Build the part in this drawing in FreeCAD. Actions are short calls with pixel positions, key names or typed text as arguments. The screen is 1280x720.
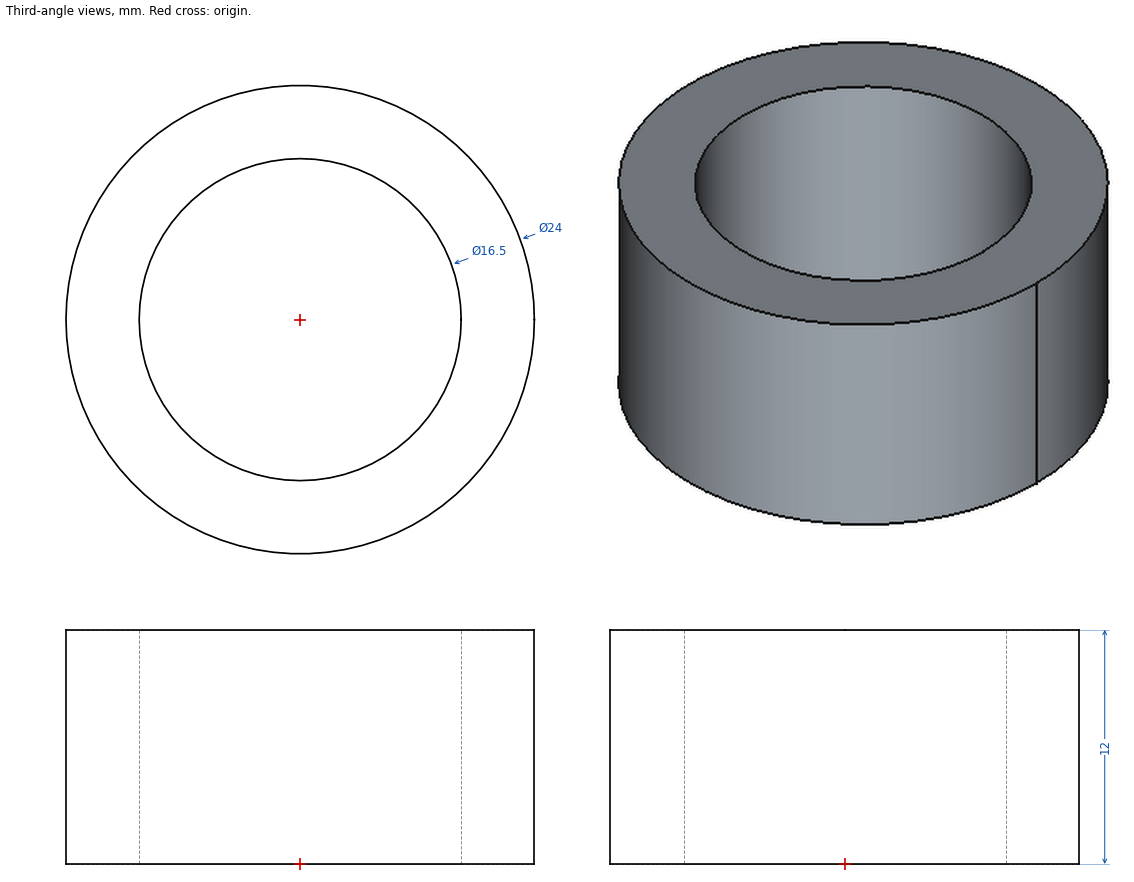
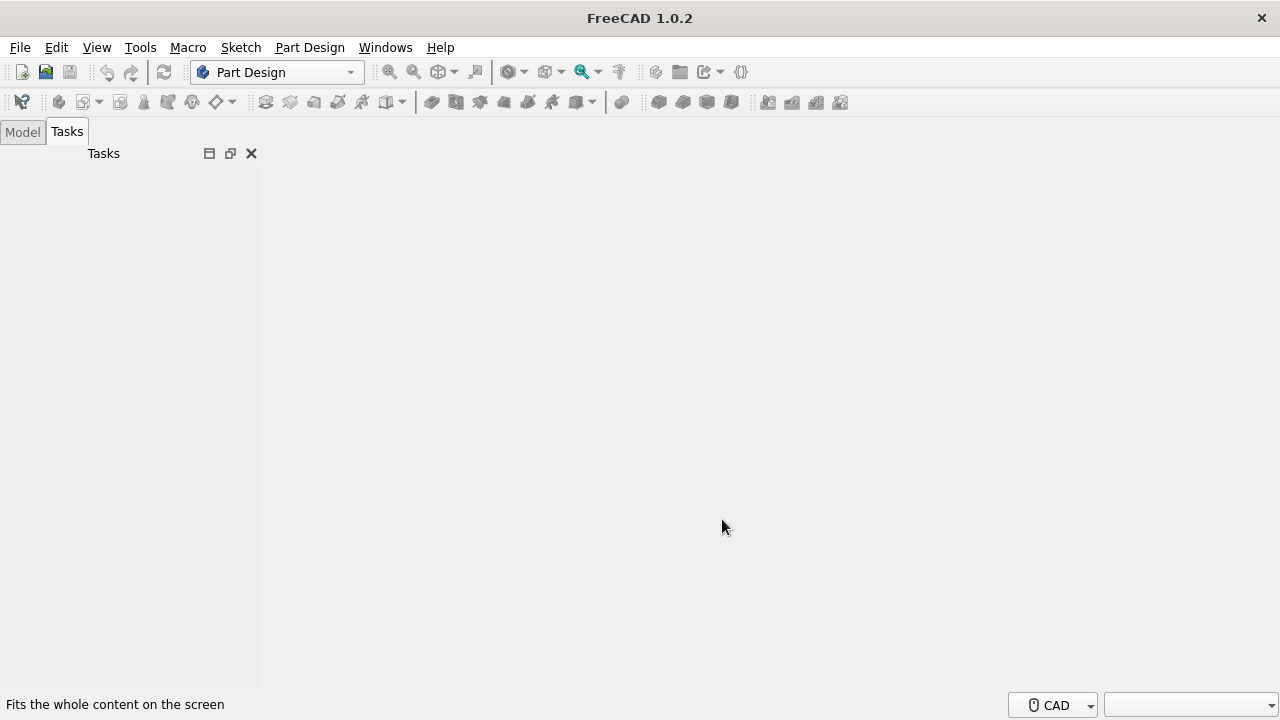
click(22, 72)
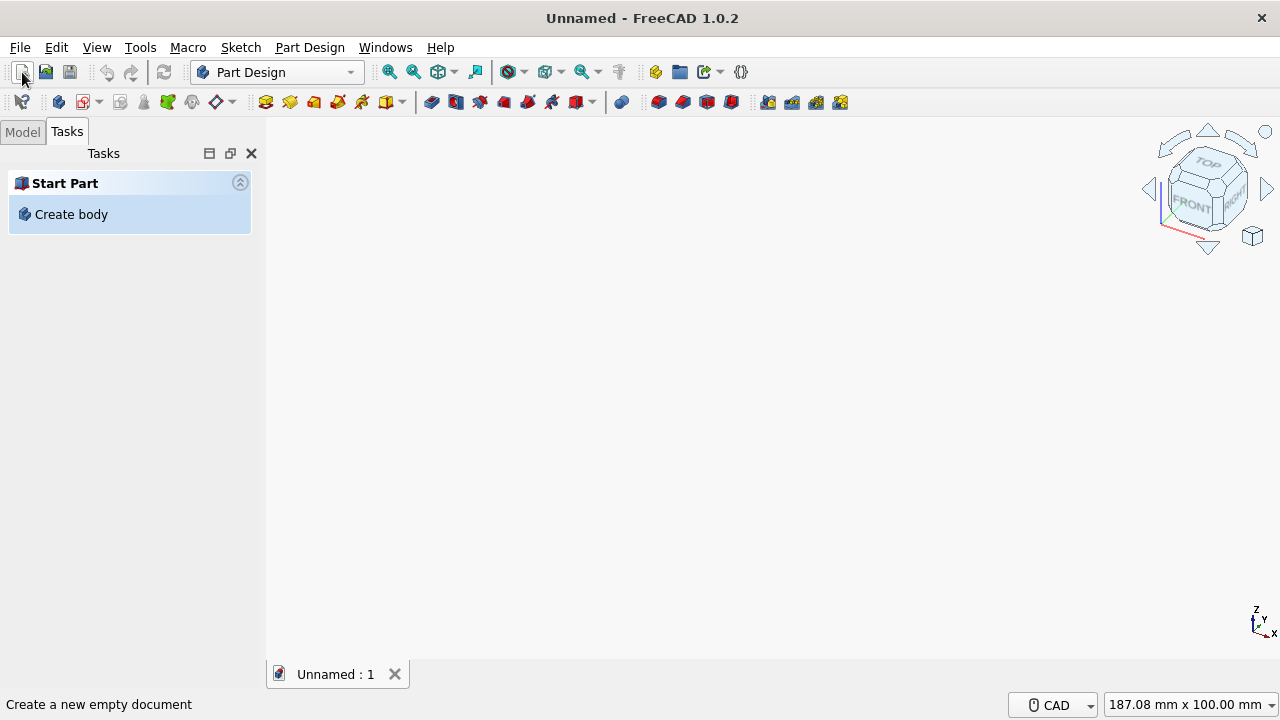
click(84, 102)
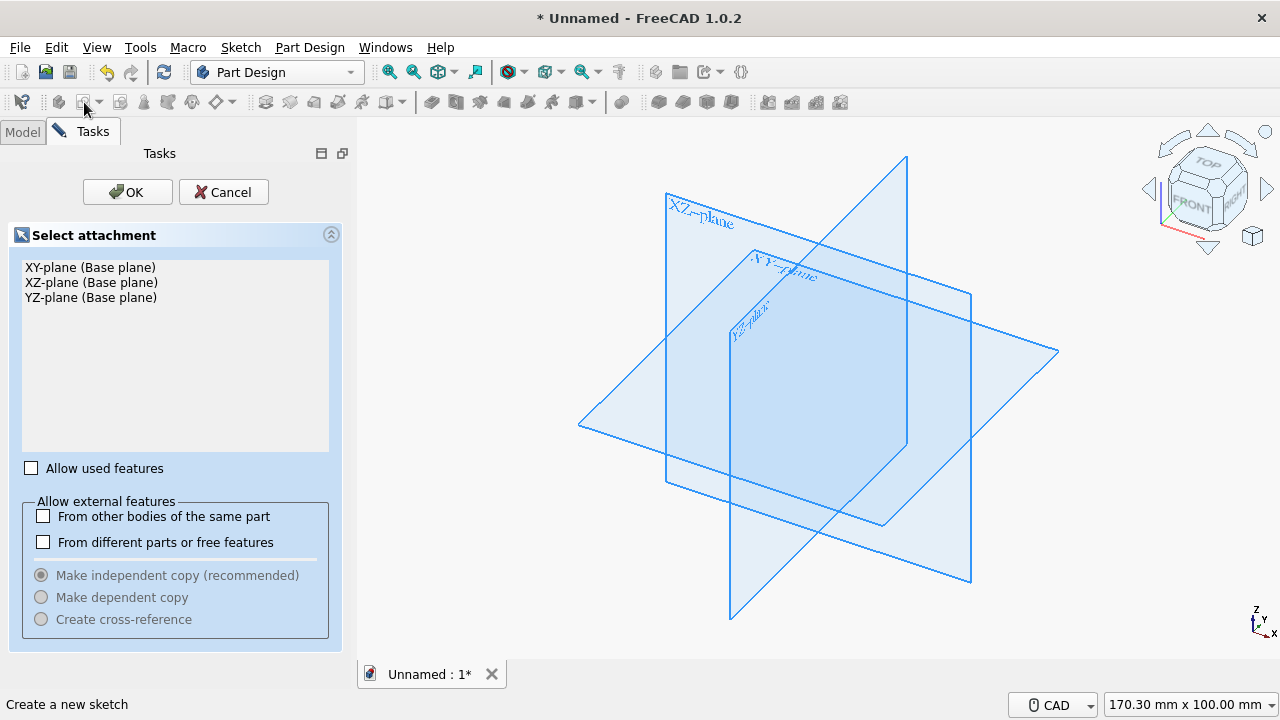
click(82, 268)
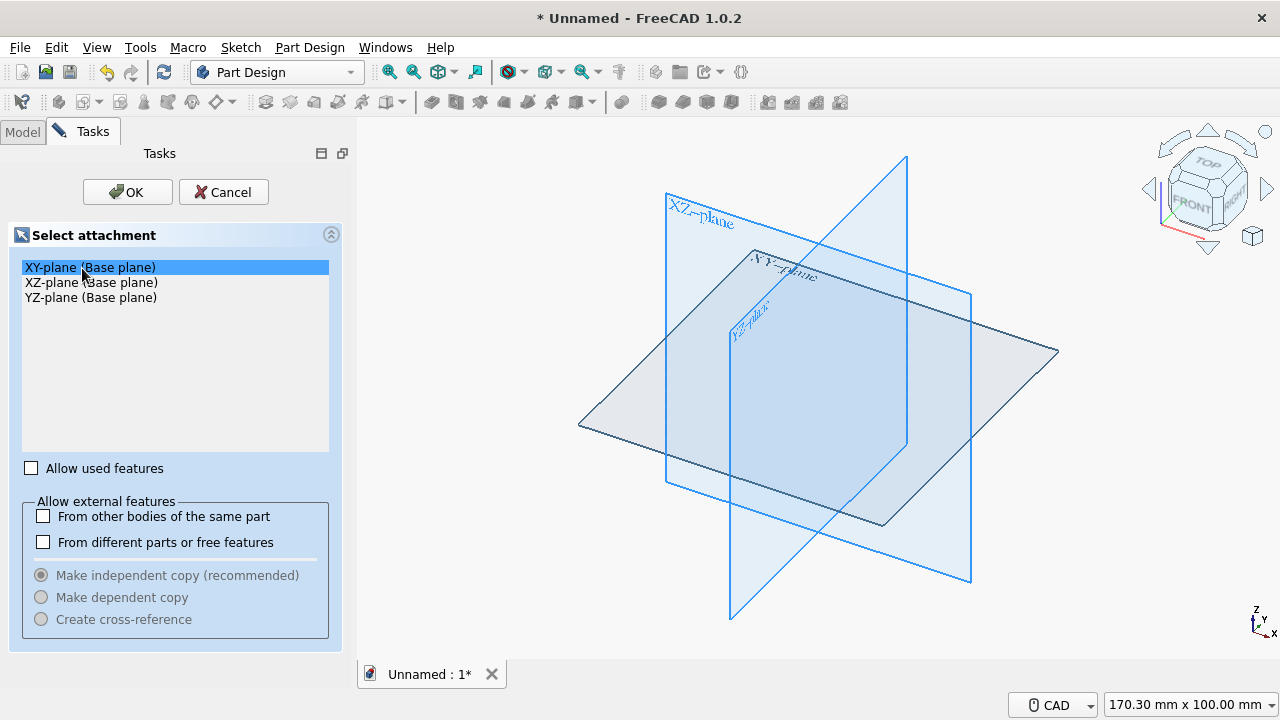
click(128, 192)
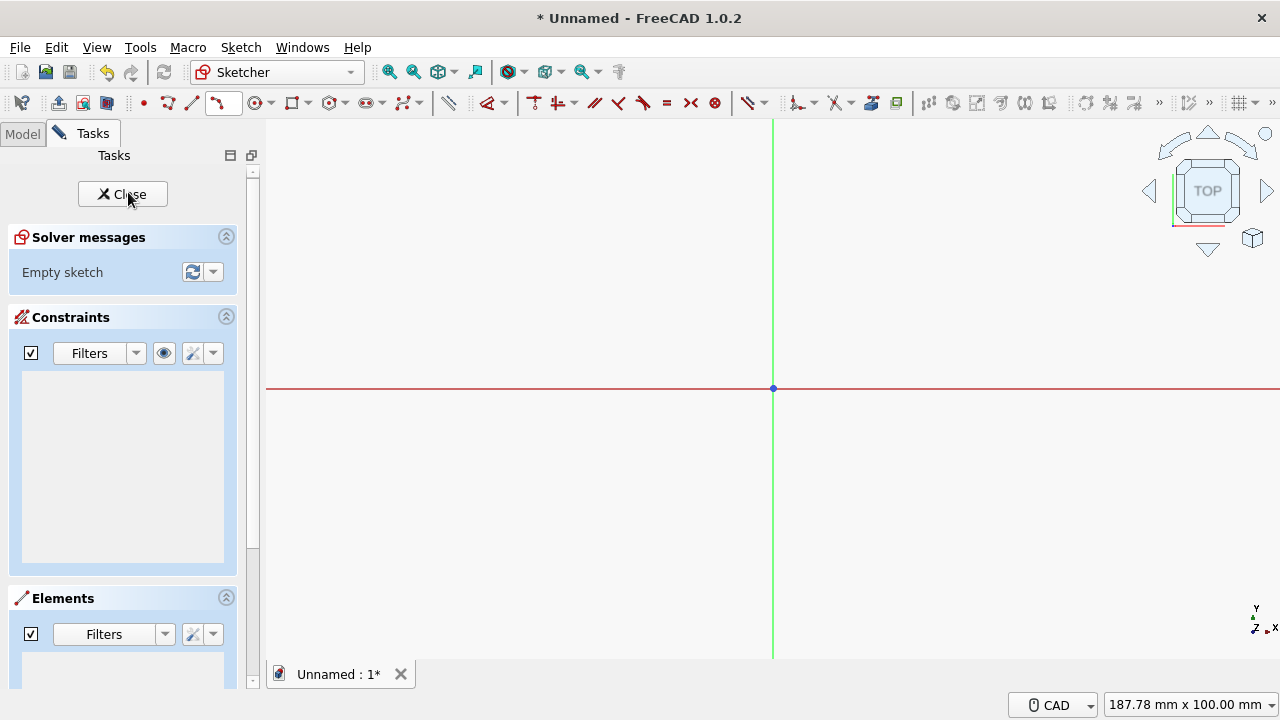
scroll(813, 389, up, 5)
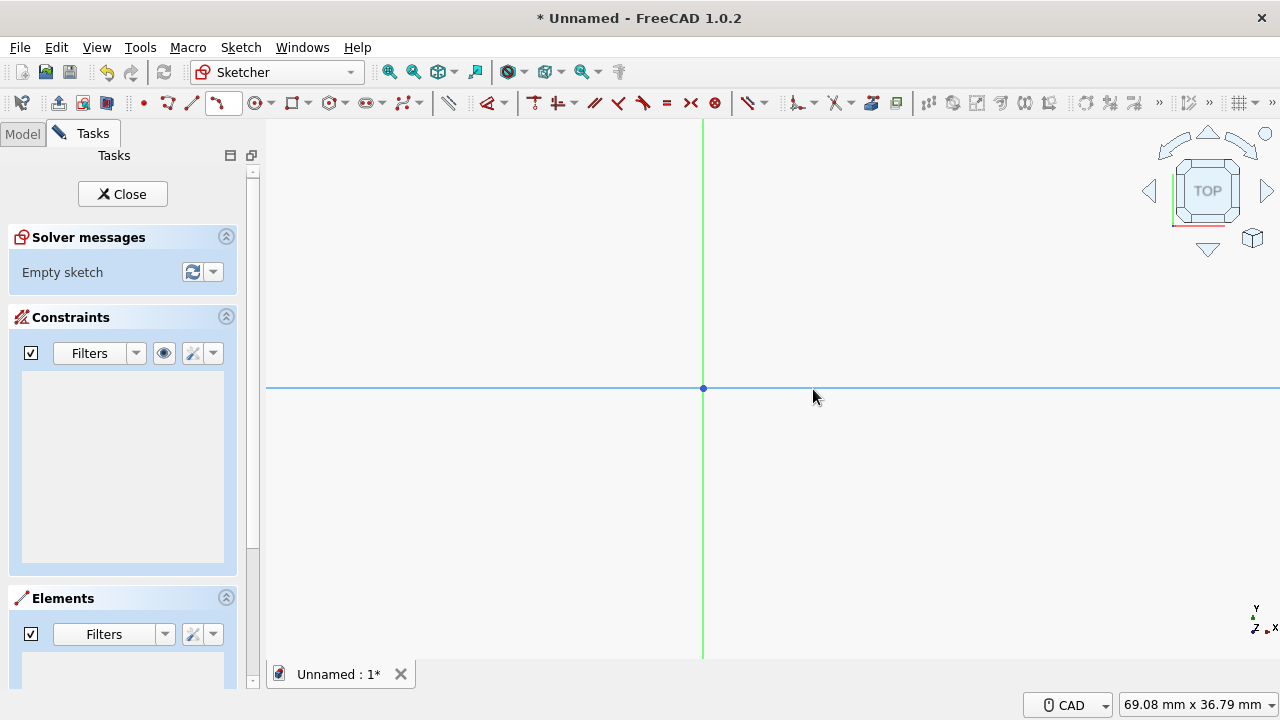
key(g)
key(c)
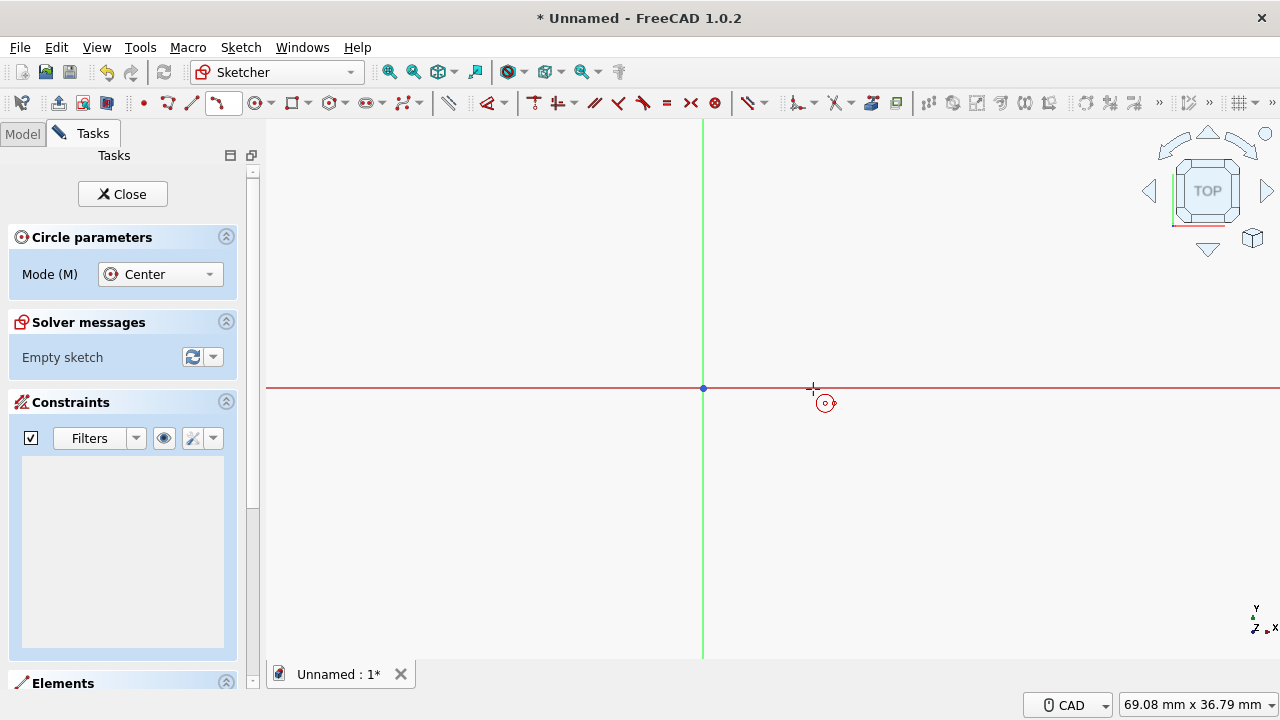
click(703, 388)
click(828, 264)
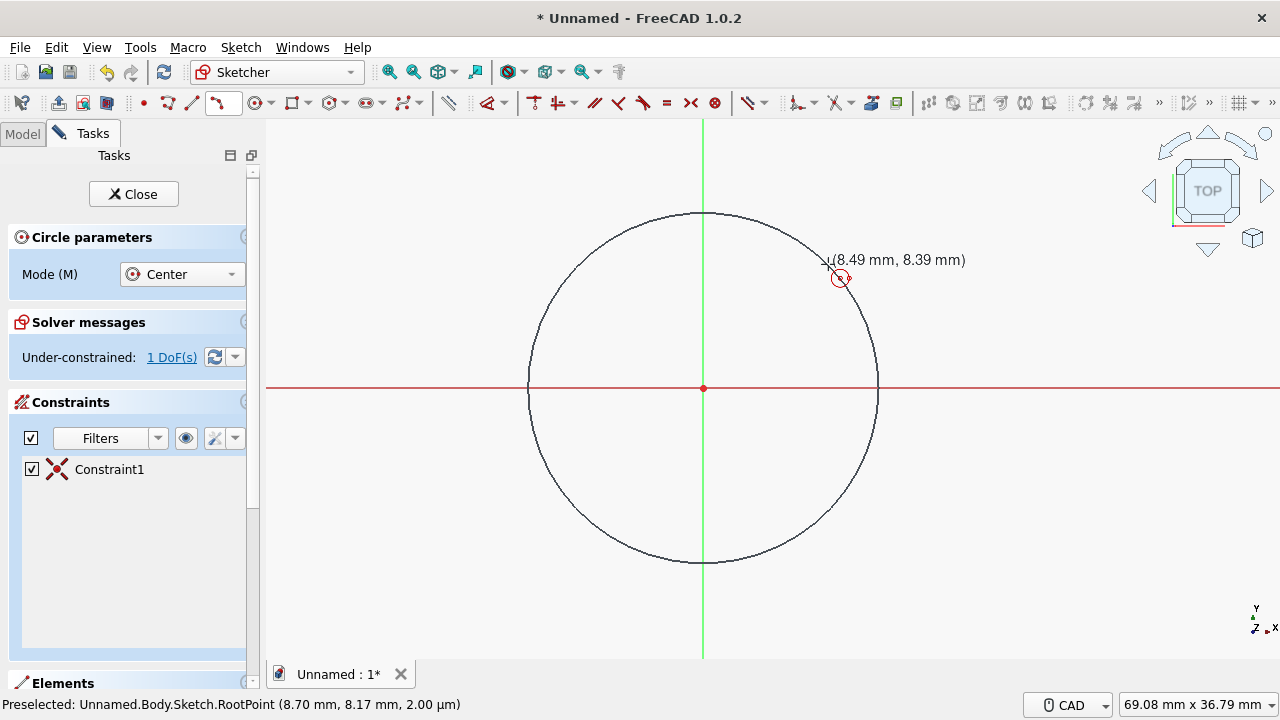
click(703, 388)
click(789, 303)
key(Escape)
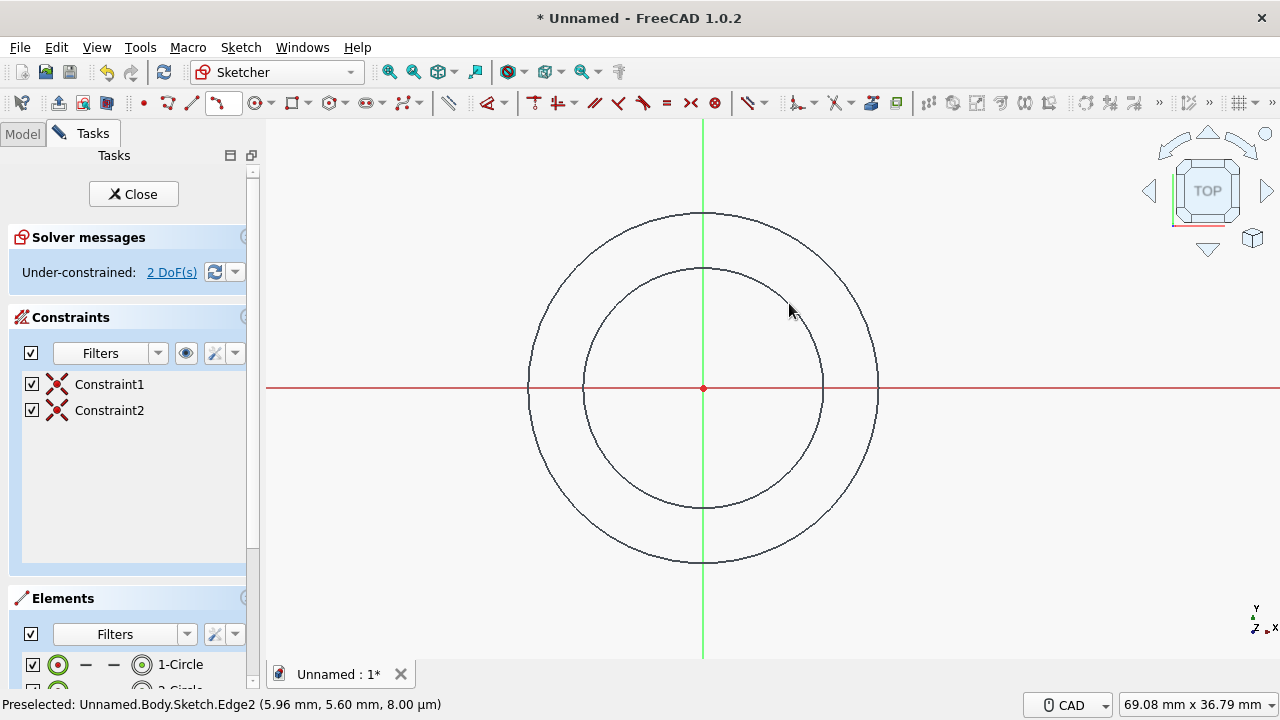
click(827, 264)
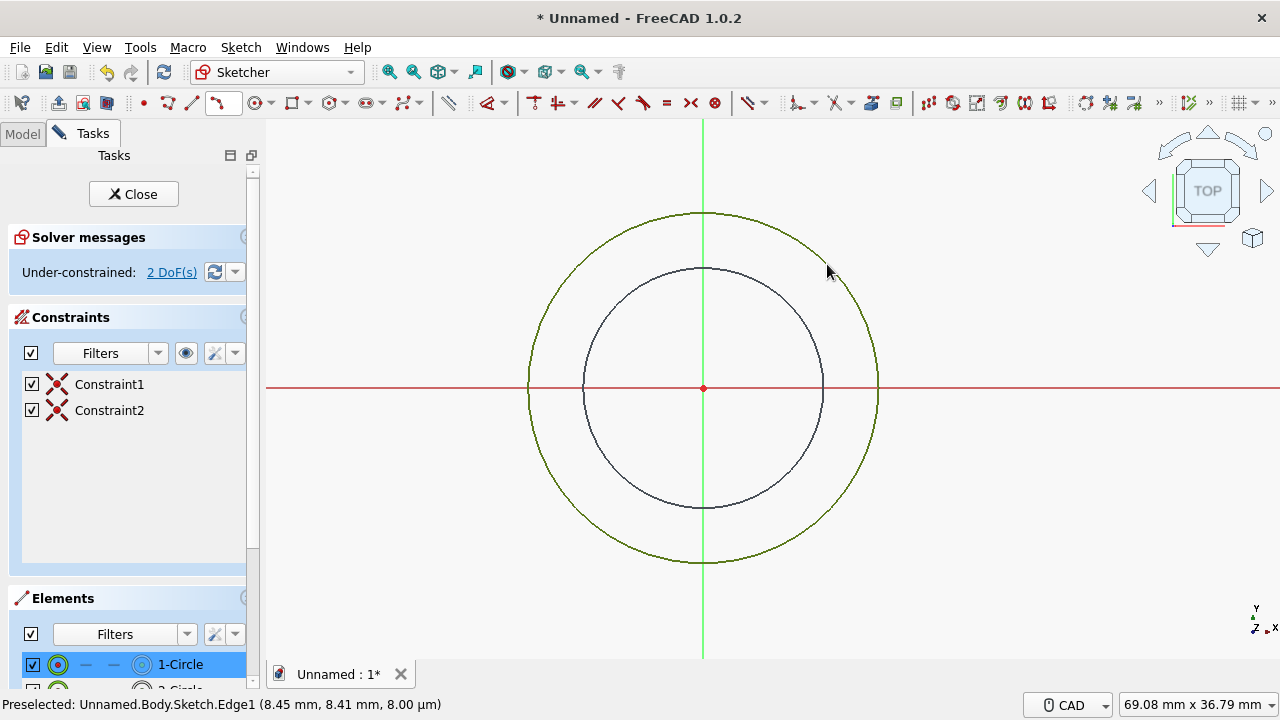
key(k)
key(o)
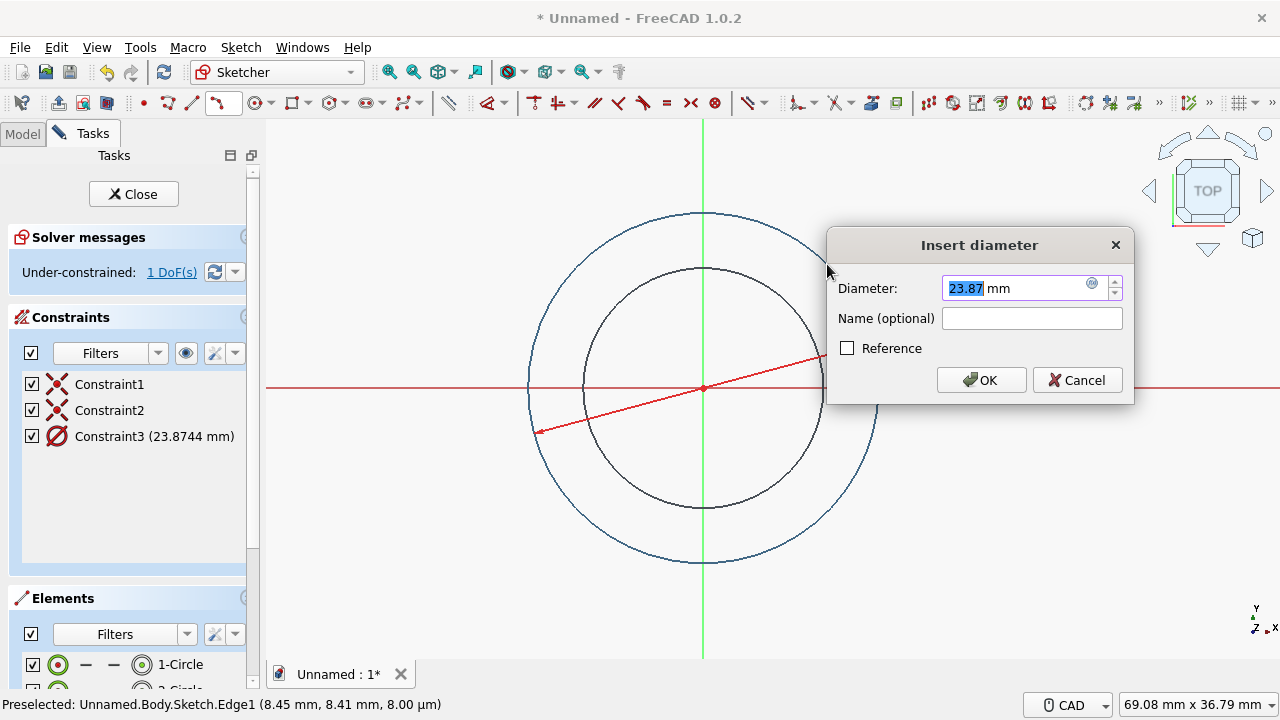
text(24)
key(Return)